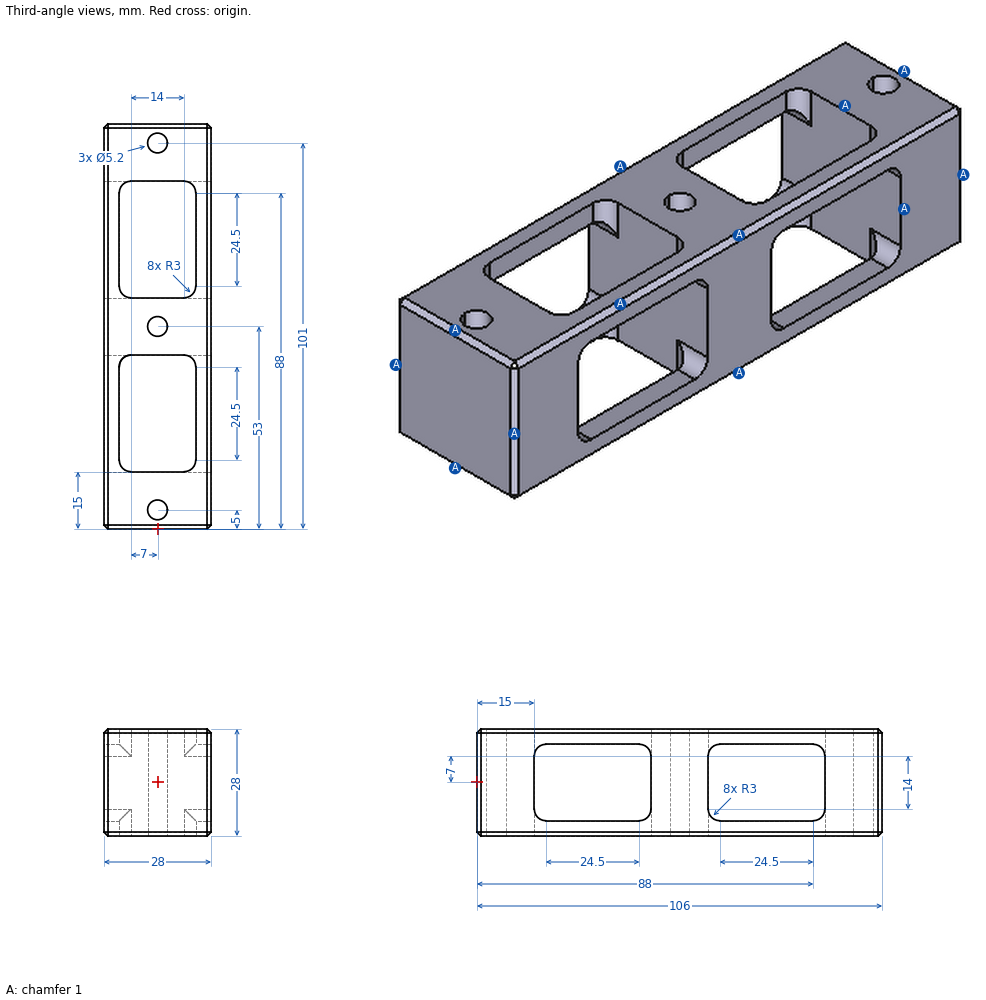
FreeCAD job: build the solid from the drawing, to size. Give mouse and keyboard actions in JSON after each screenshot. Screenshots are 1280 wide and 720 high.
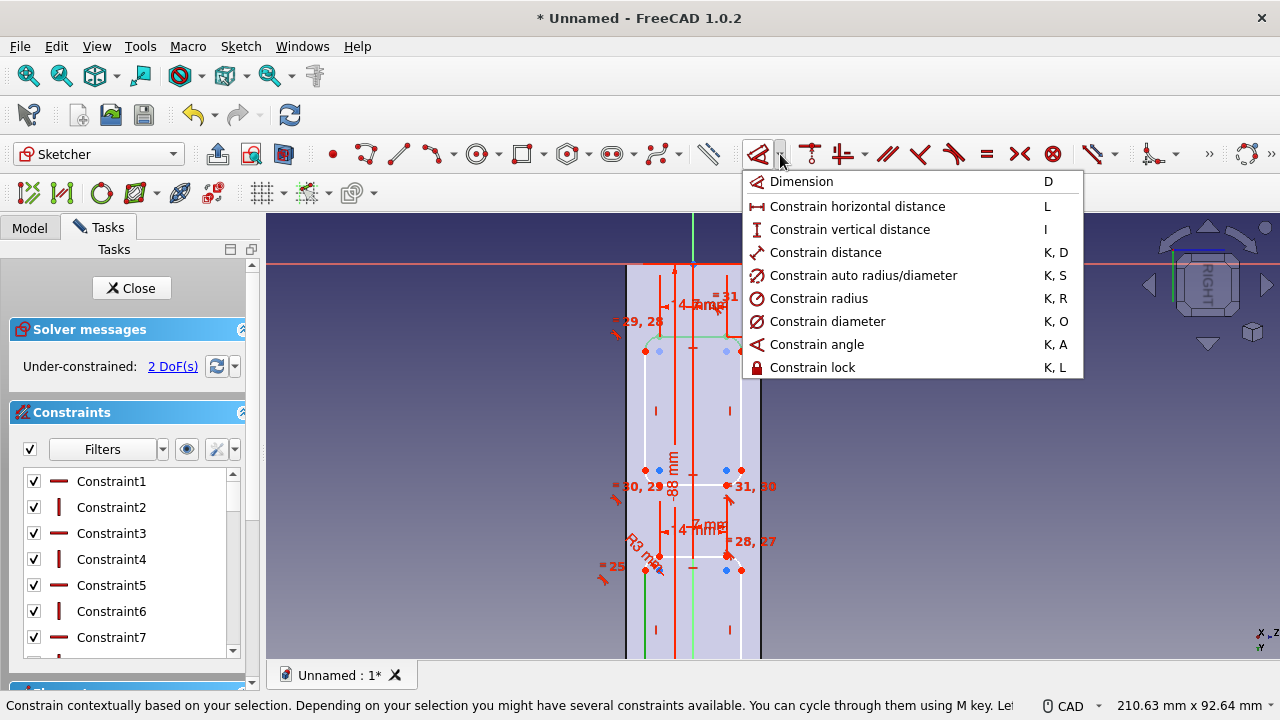
{"action": "left_click", "coordinate": [913, 230]}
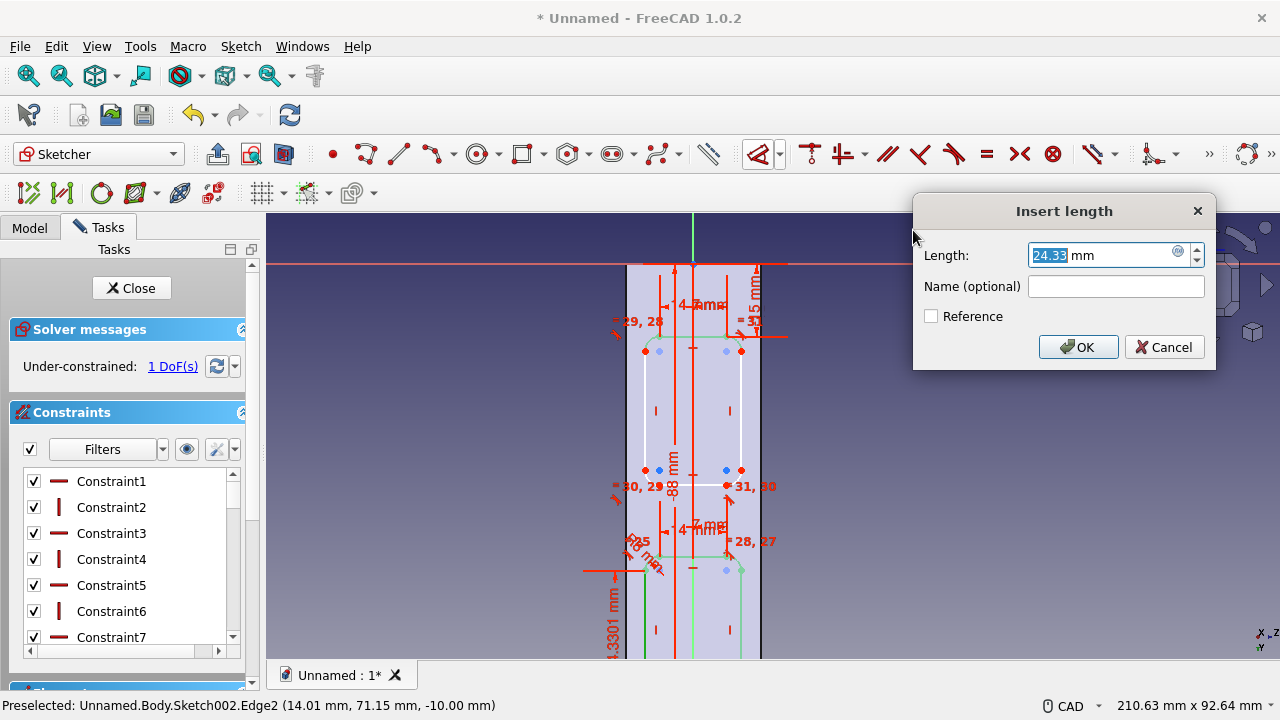
{"action": "type", "text": "24.5"}
{"action": "key", "text": "Return"}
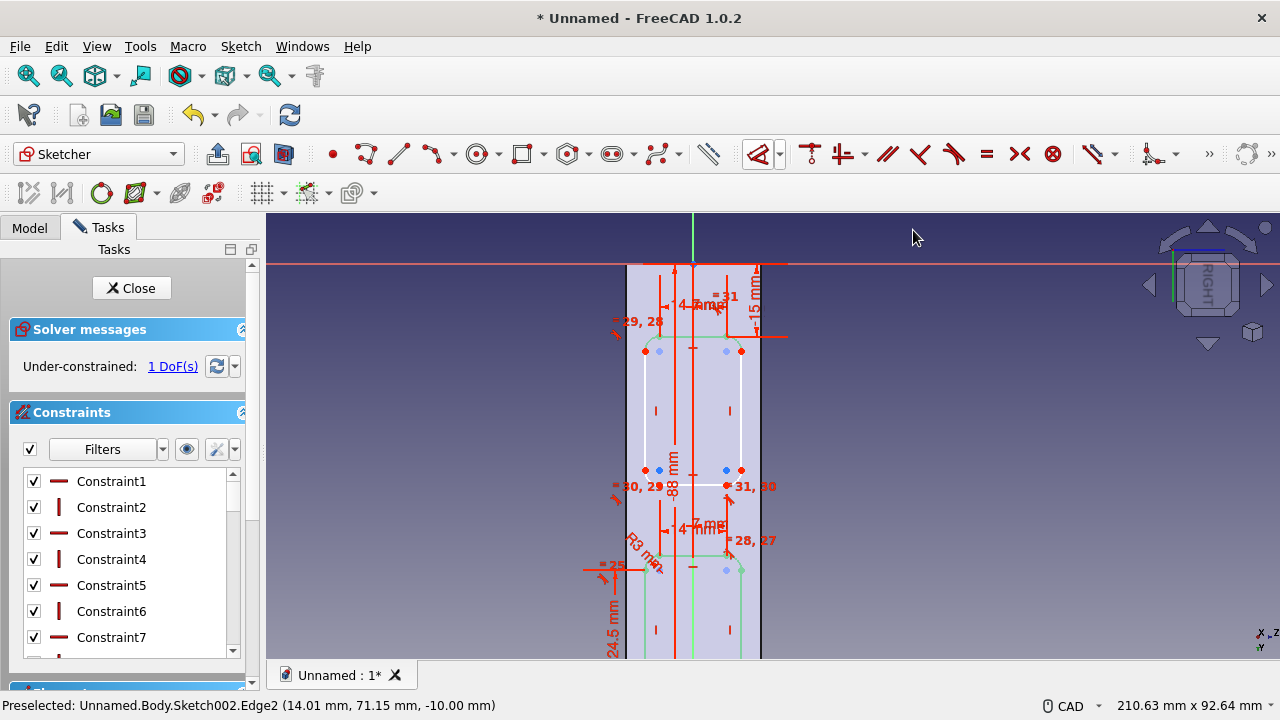
{"action": "left_click", "coordinate": [645, 387]}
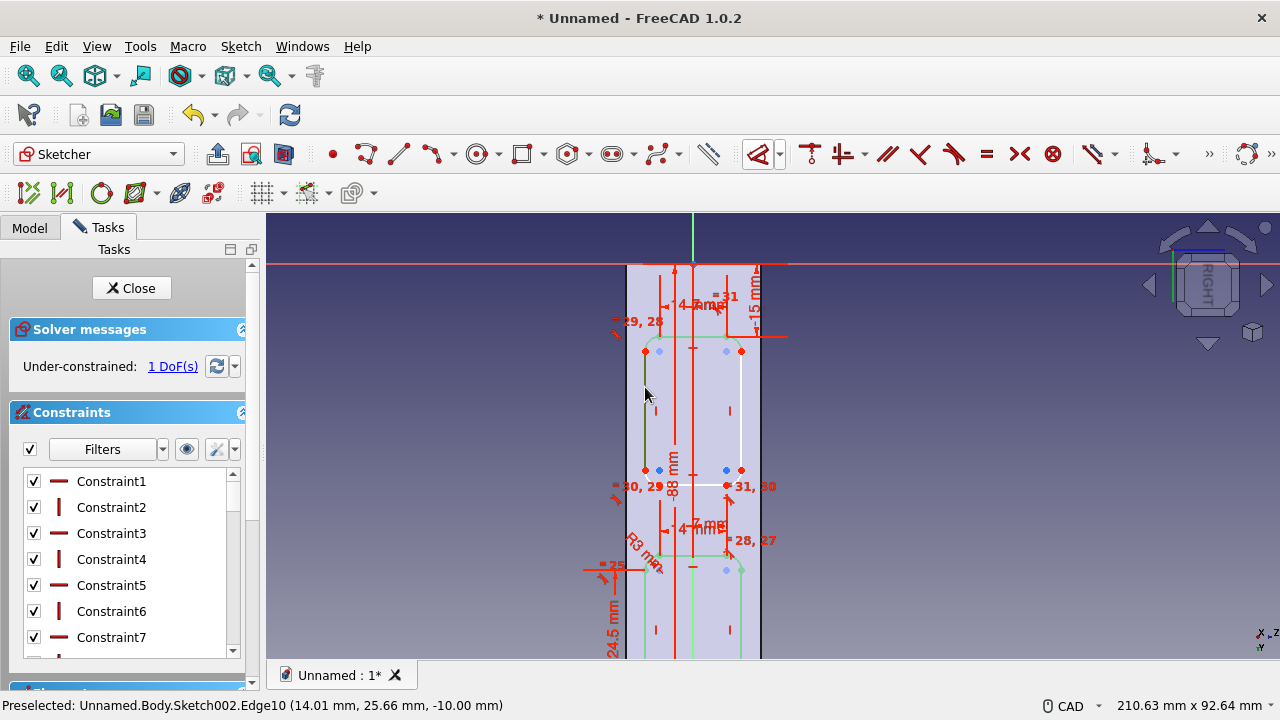
{"action": "key", "text": "i"}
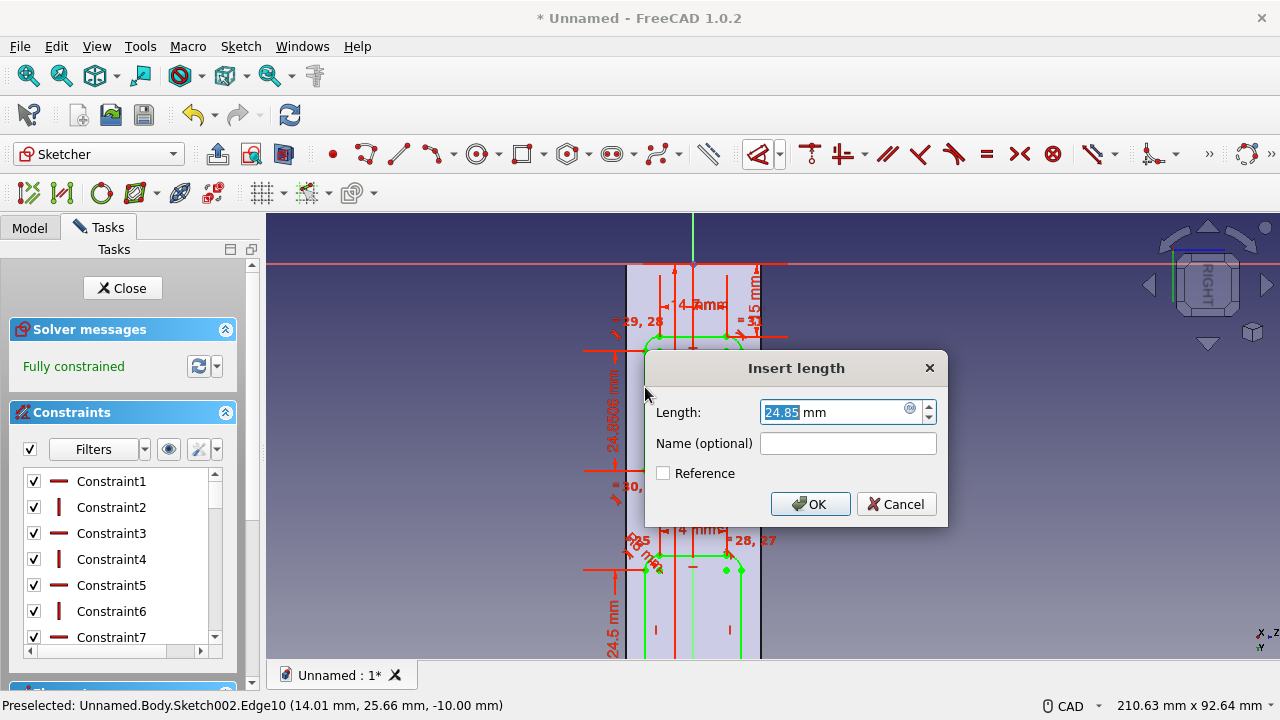
{"action": "type", "text": "24.5"}
{"action": "key", "text": "Return"}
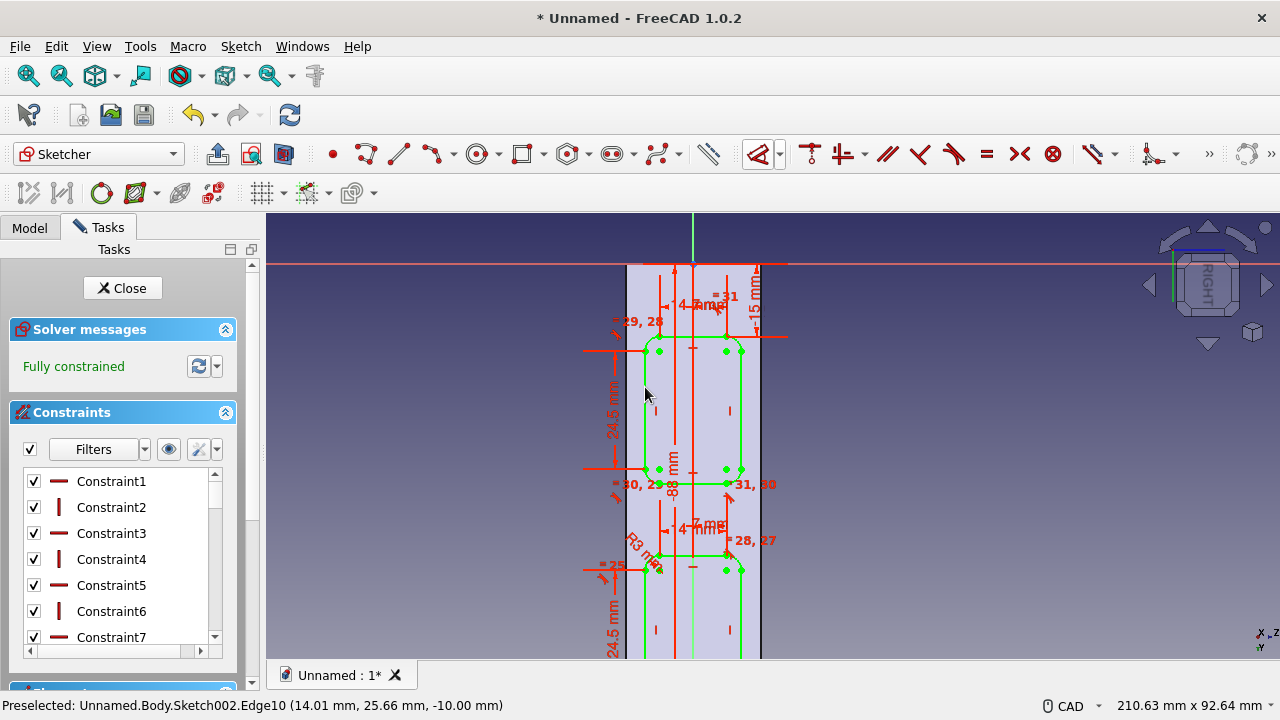
{"action": "left_click", "coordinate": [123, 288]}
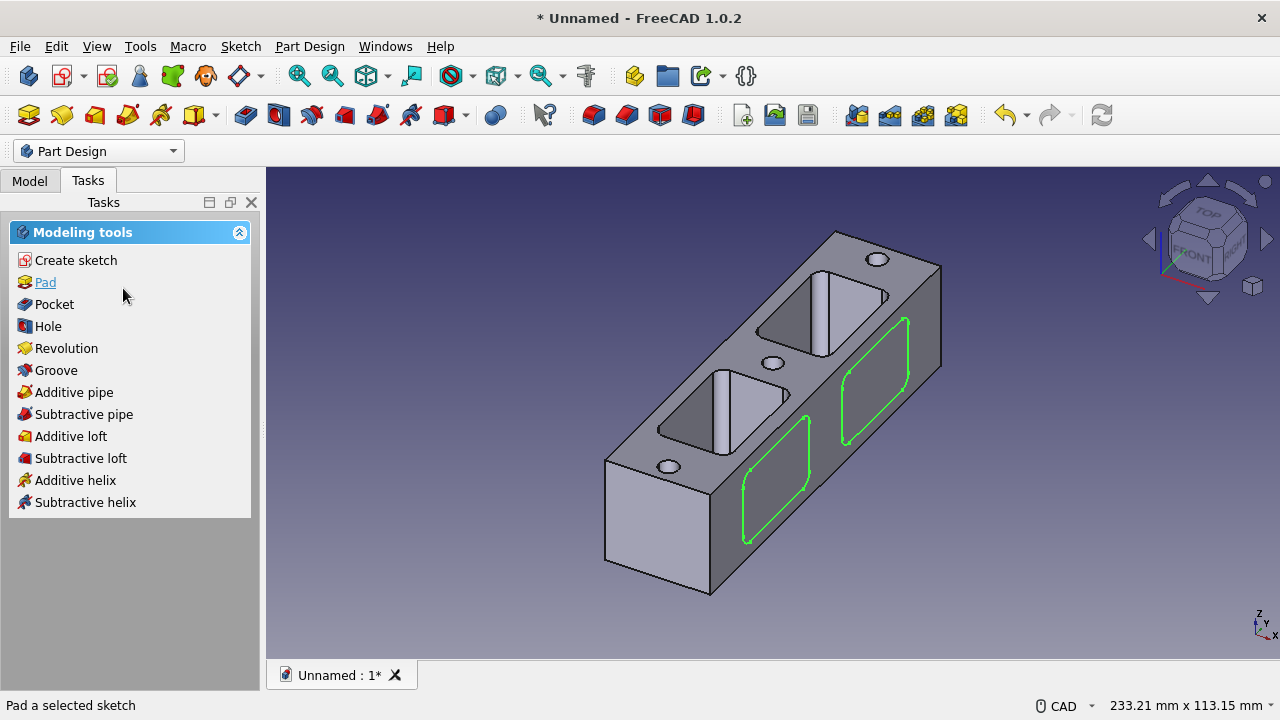
{"action": "left_click", "coordinate": [246, 116]}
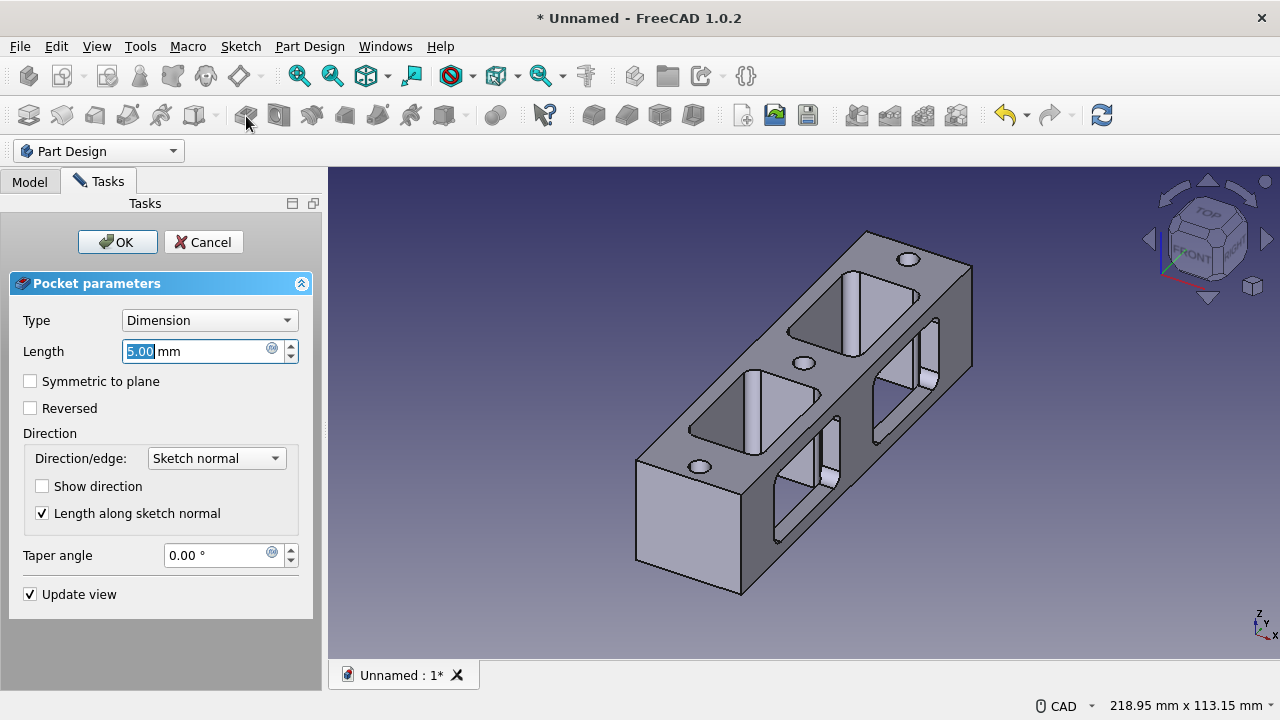
{"action": "left_click", "coordinate": [210, 320]}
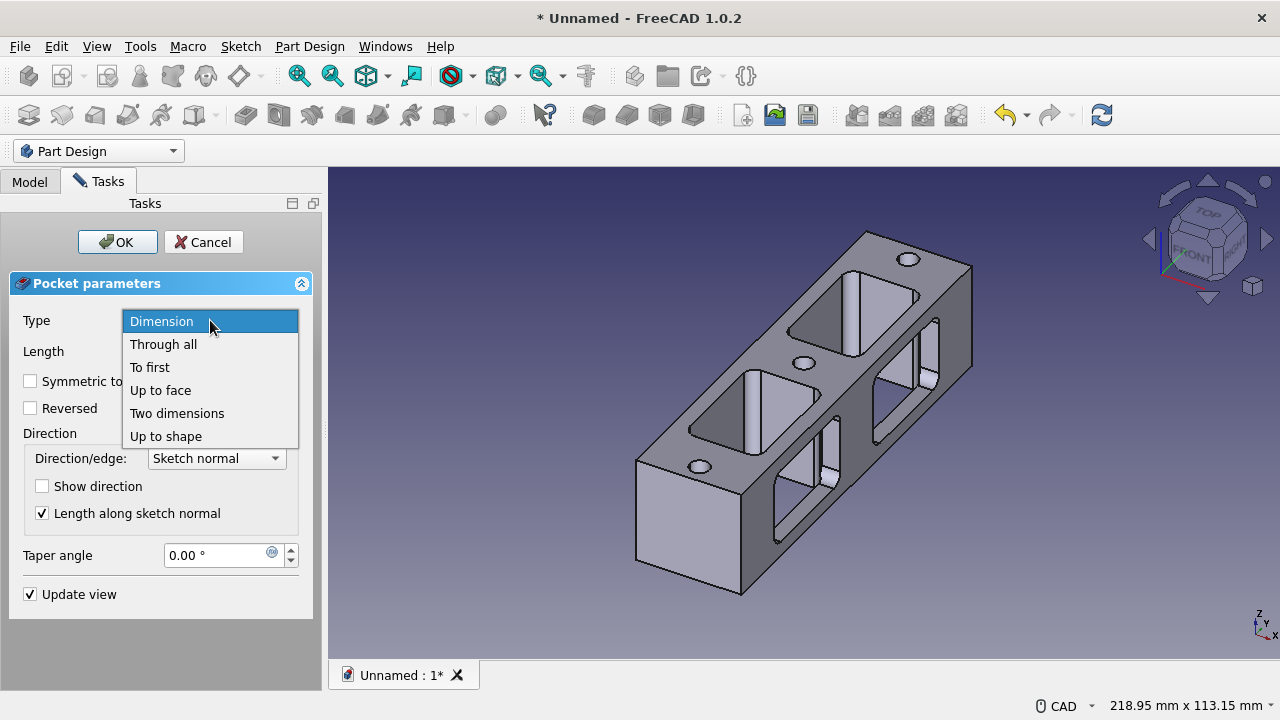
{"action": "left_click", "coordinate": [208, 344]}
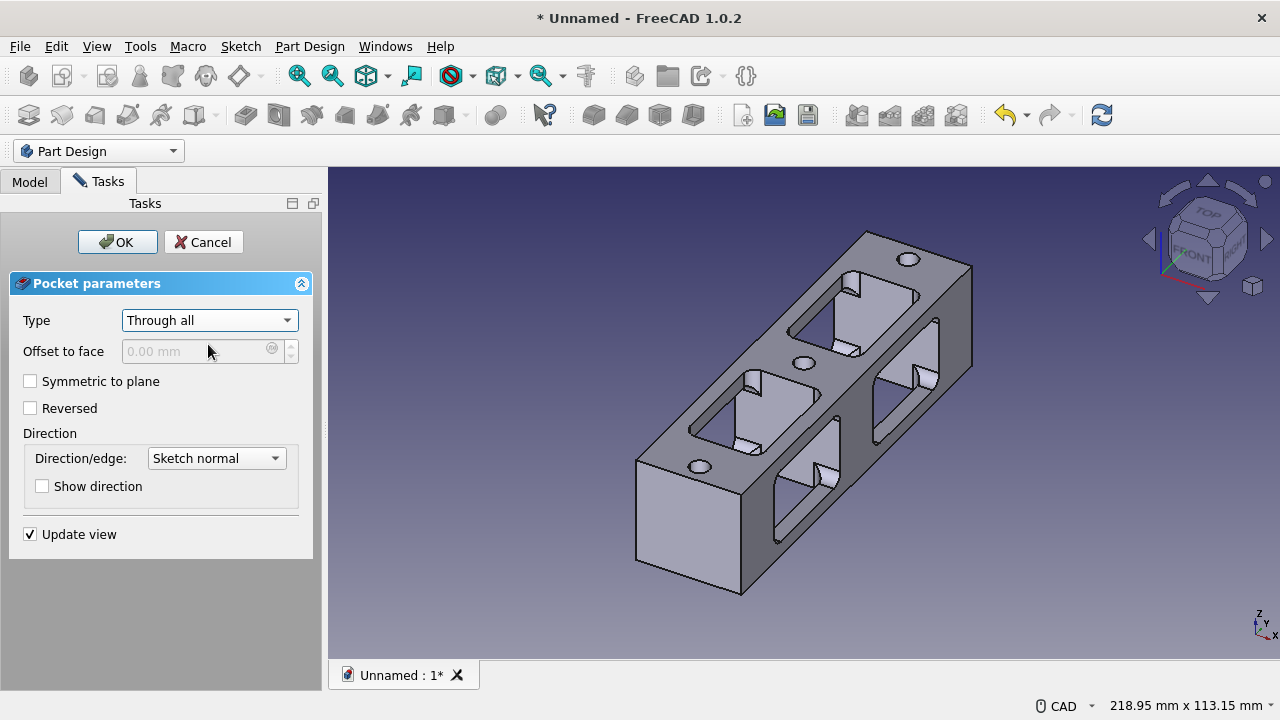
{"action": "left_click", "coordinate": [118, 242]}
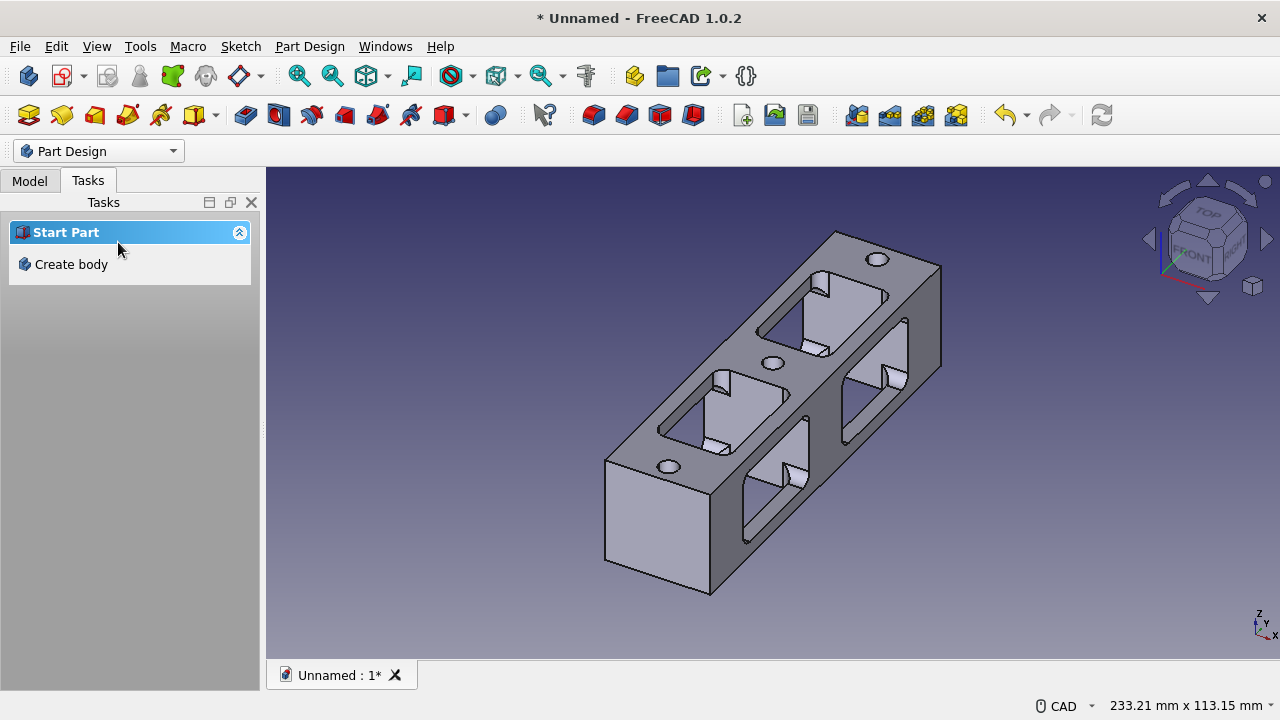
{"action": "left_click", "coordinate": [658, 526]}